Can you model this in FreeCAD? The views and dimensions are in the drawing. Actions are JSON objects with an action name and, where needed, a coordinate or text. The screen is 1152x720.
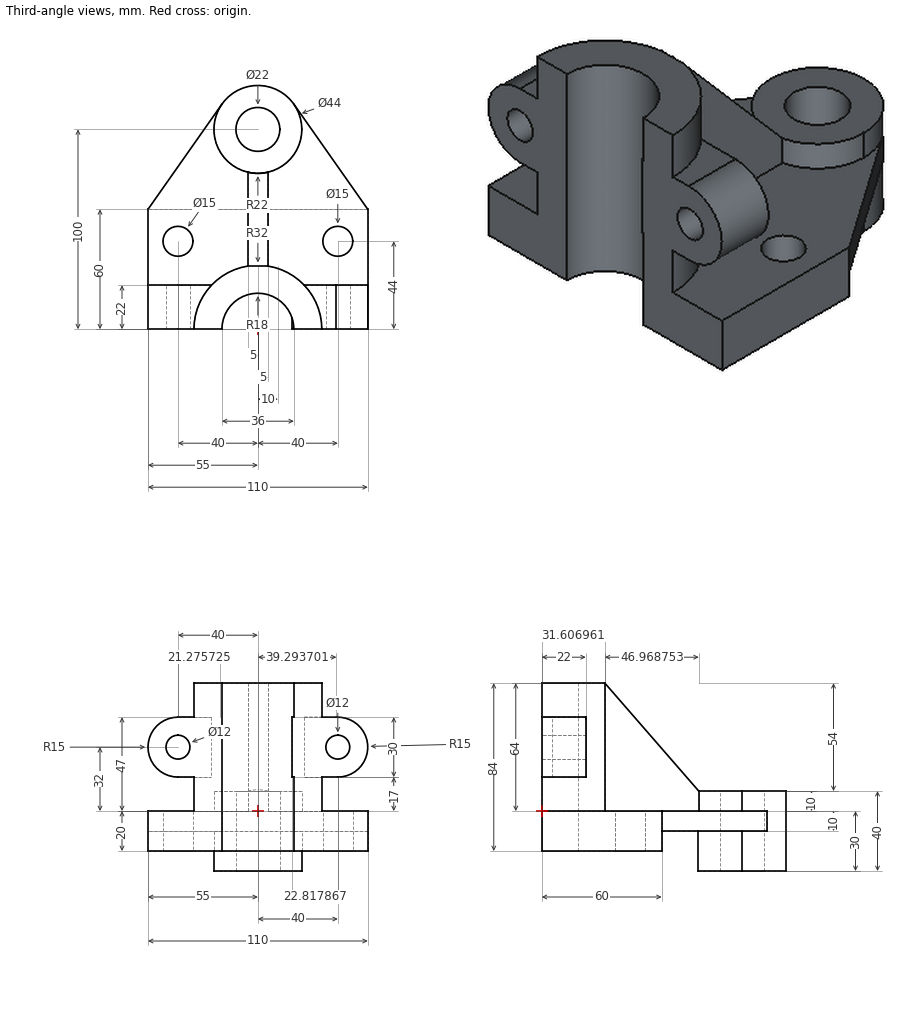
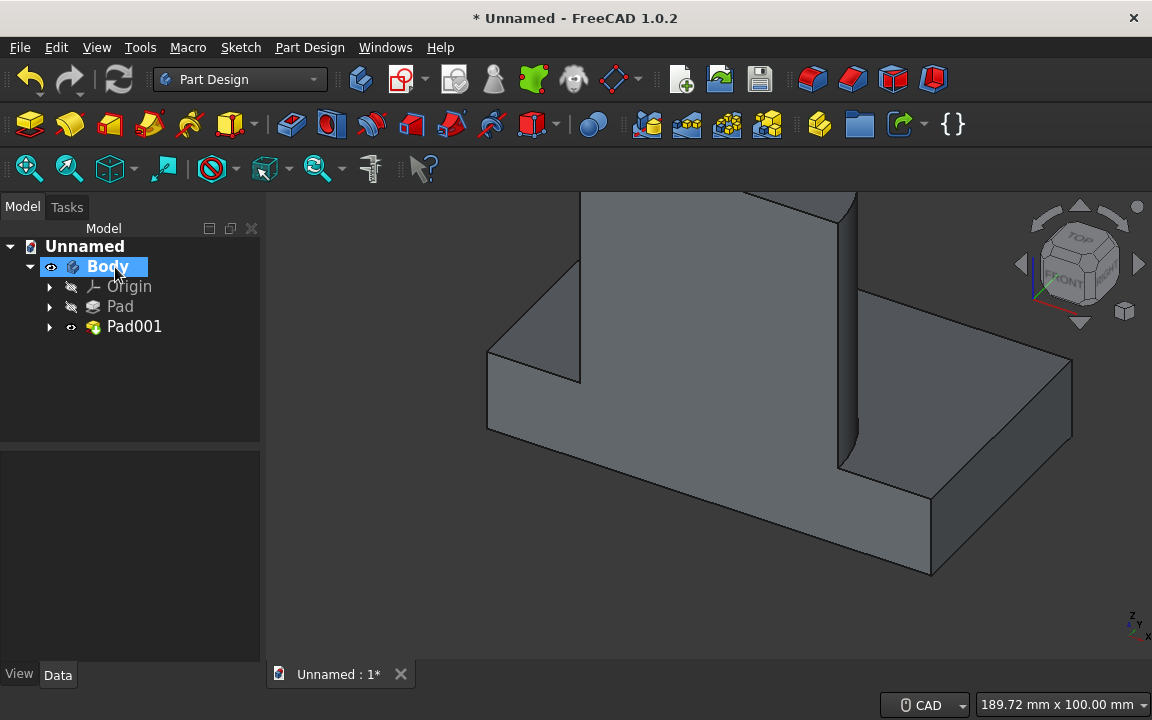
{"action": "left_click", "coordinate": [30, 170]}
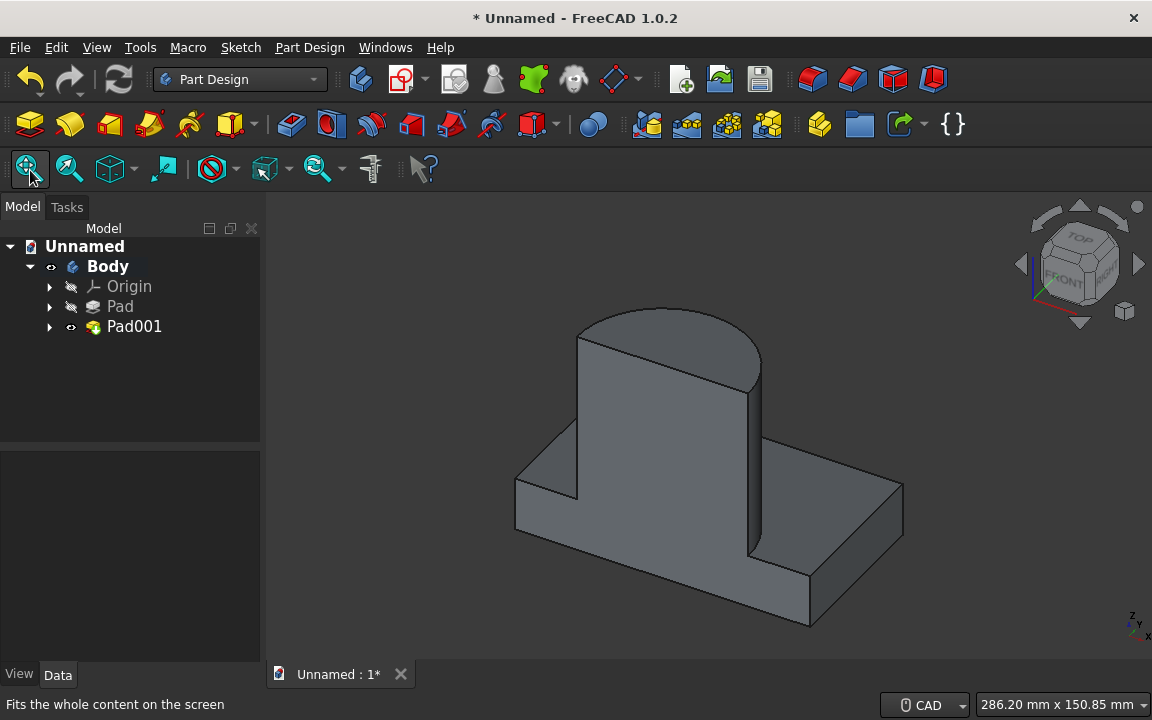
{"action": "left_click", "coordinate": [687, 340]}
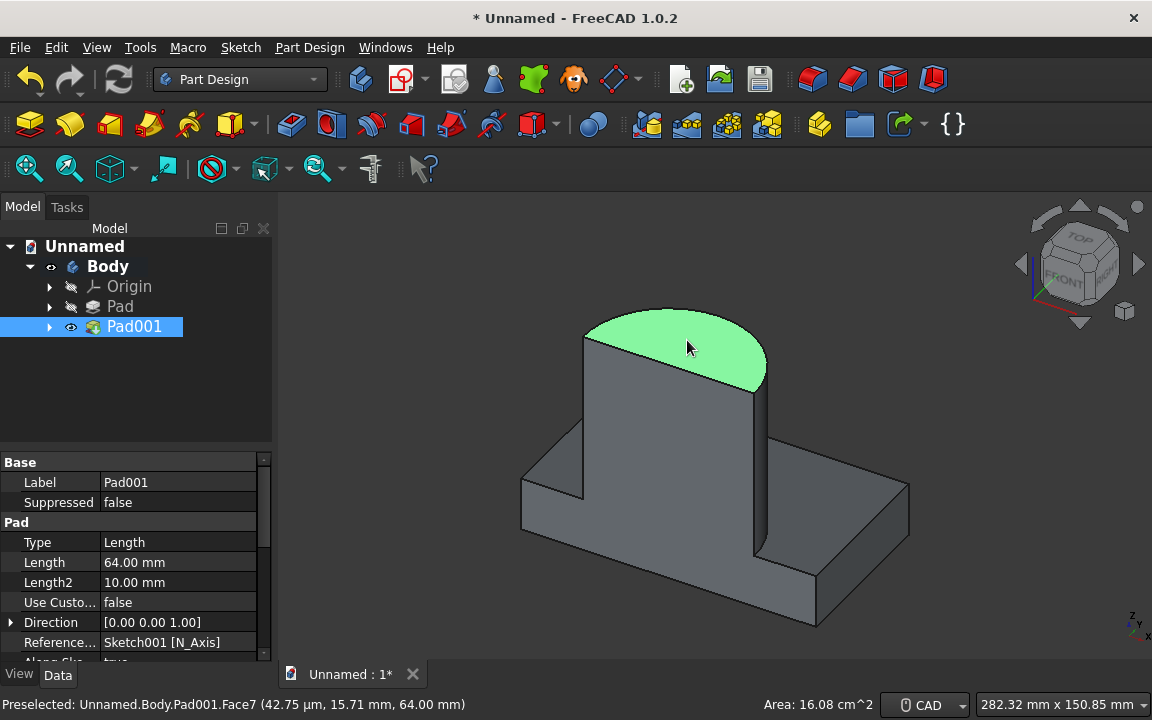
{"action": "left_click", "coordinate": [402, 80]}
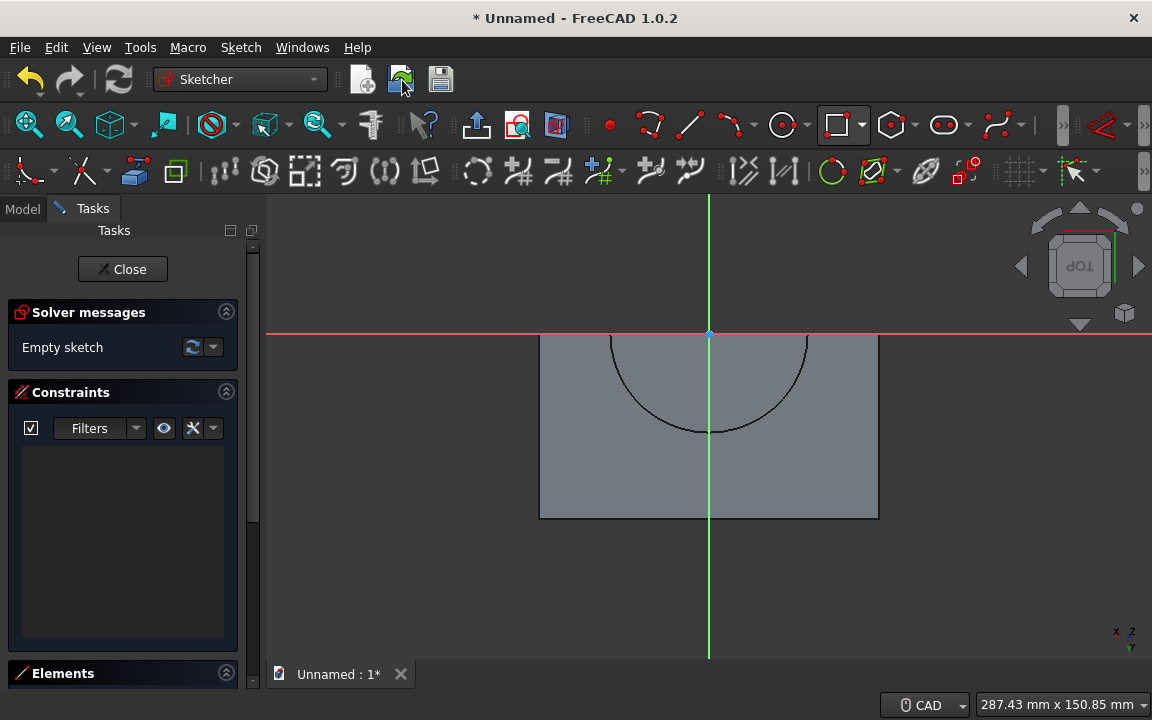
{"action": "scroll", "coordinate": [731, 341], "scroll_direction": "up", "scroll_amount": 7}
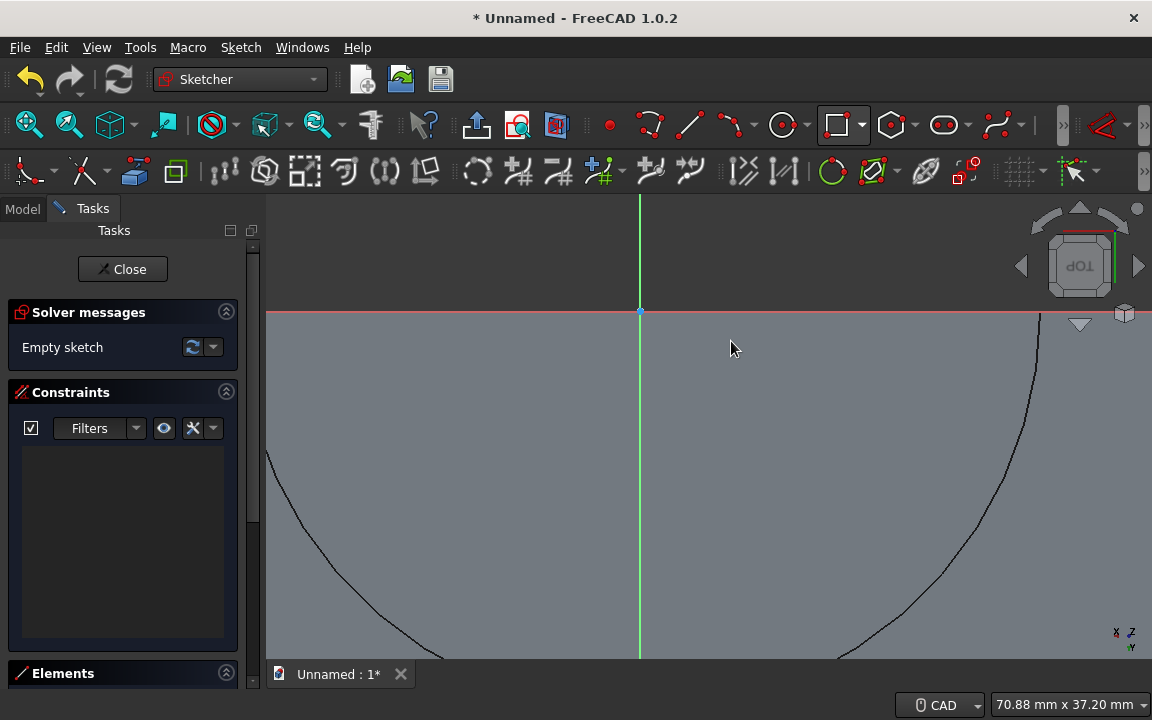
{"action": "left_click", "coordinate": [690, 126]}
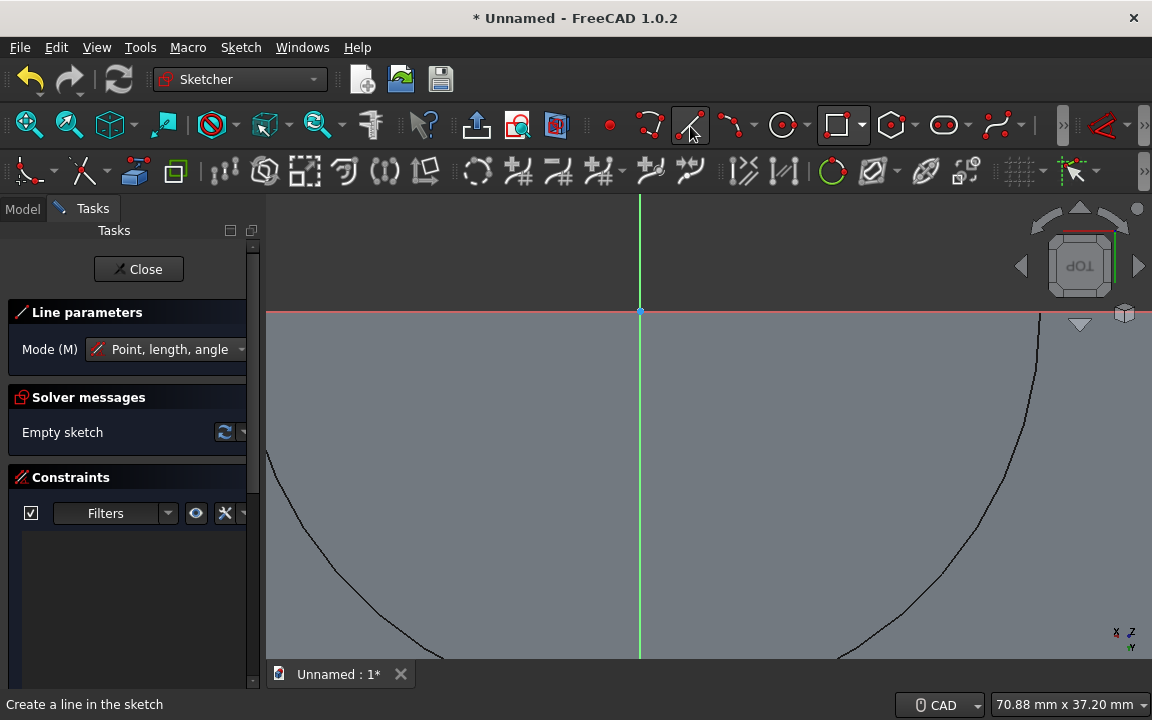
{"action": "left_click", "coordinate": [865, 312]}
{"action": "left_click", "coordinate": [415, 321]}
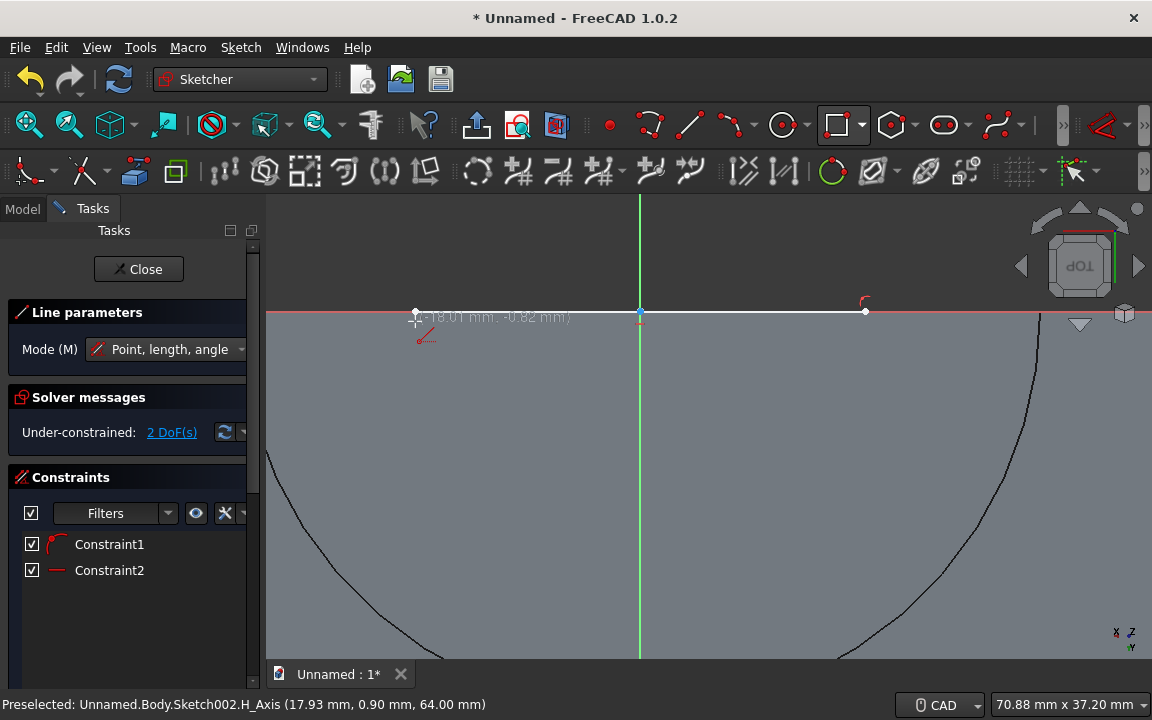
{"action": "left_click", "coordinate": [730, 126]}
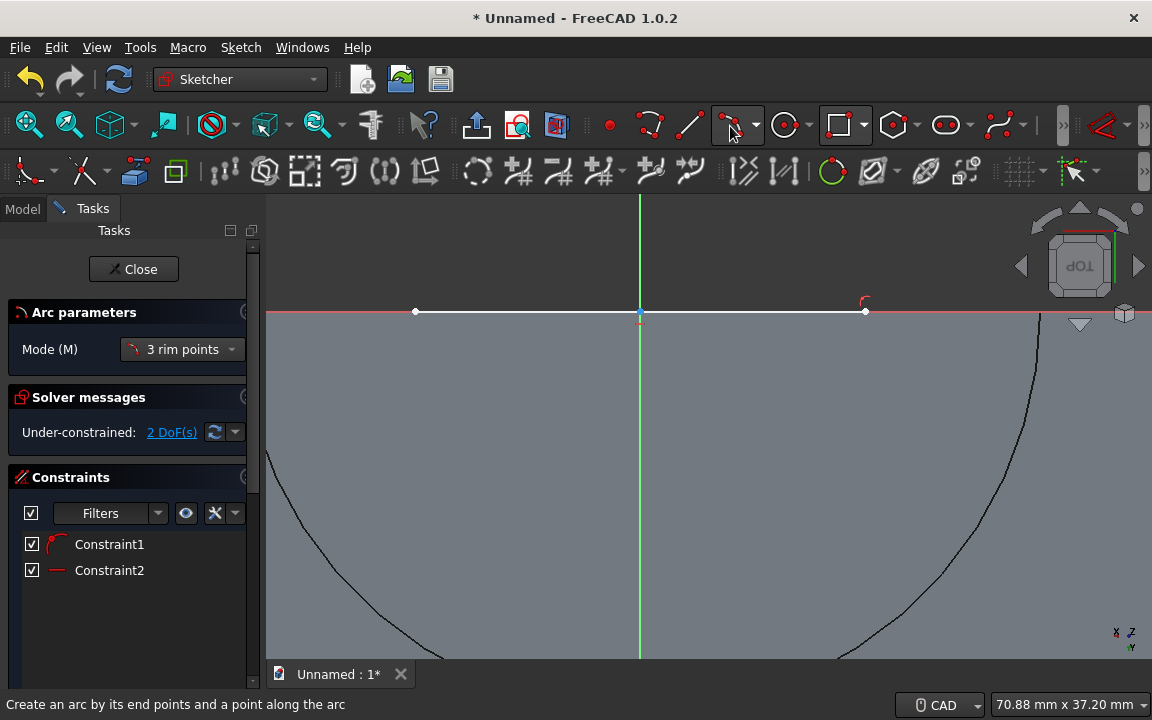
{"action": "left_click", "coordinate": [415, 321]}
{"action": "left_click", "coordinate": [865, 312]}
{"action": "left_click", "coordinate": [571, 526]}
{"action": "key", "text": "Escape"}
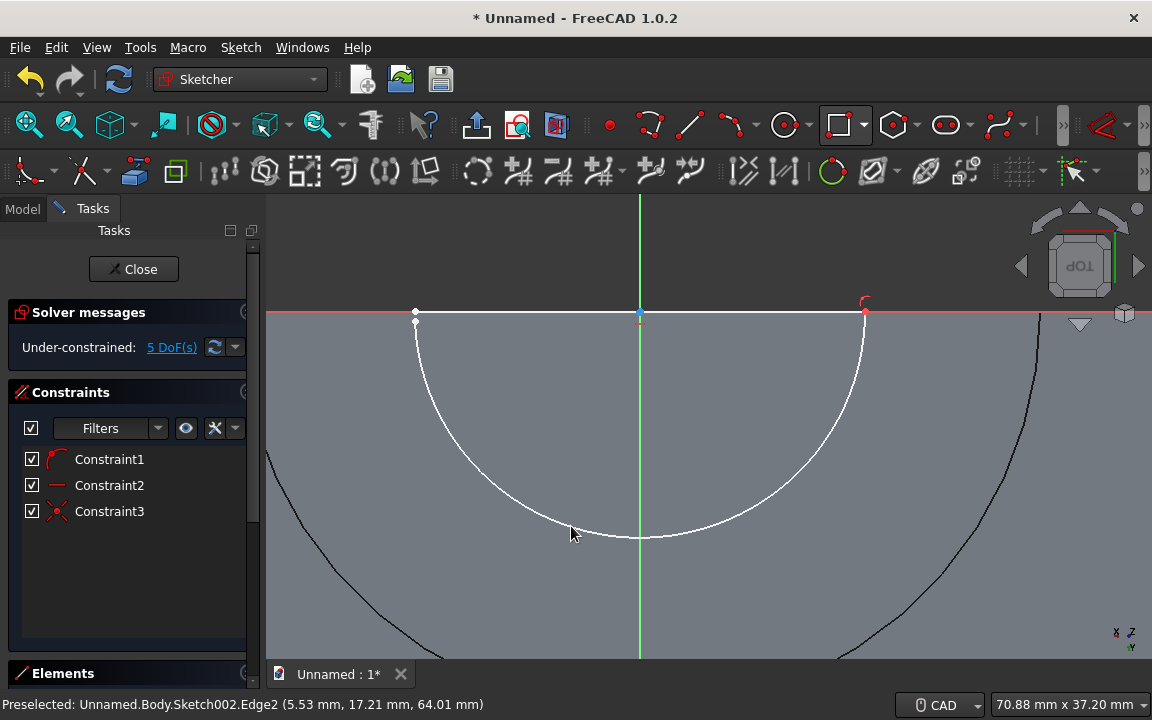
{"action": "left_click_drag", "start_coordinate": [630, 302], "coordinate": [650, 323]}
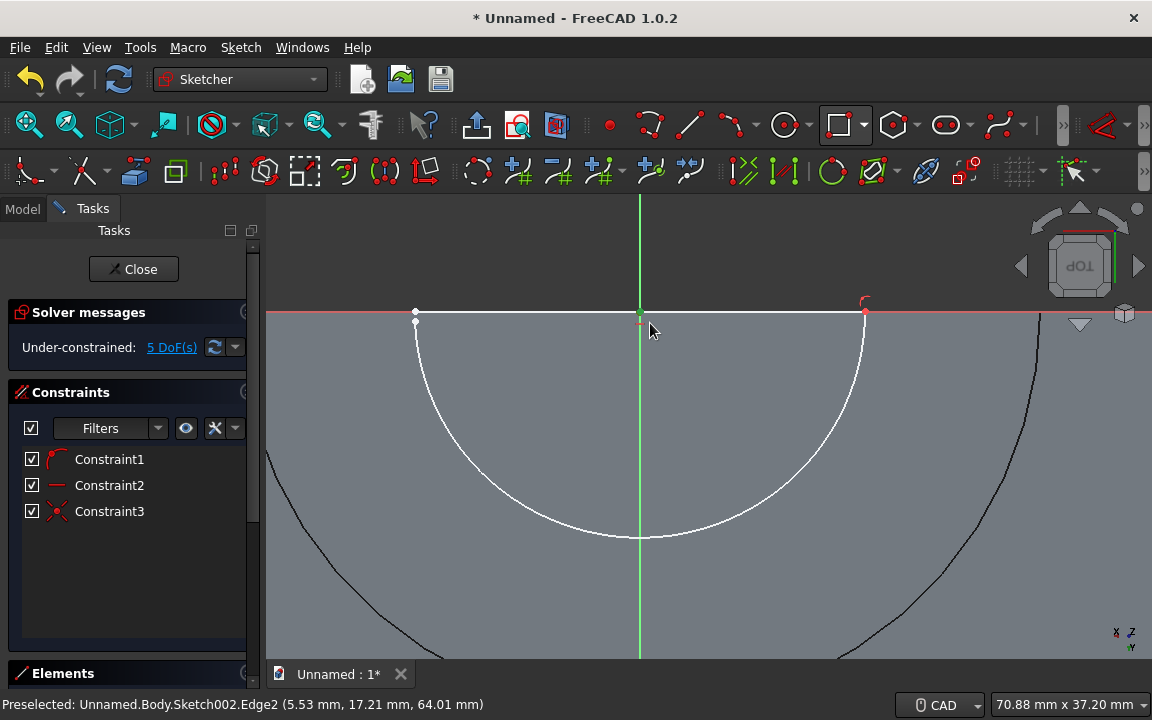
{"action": "key", "text": "c"}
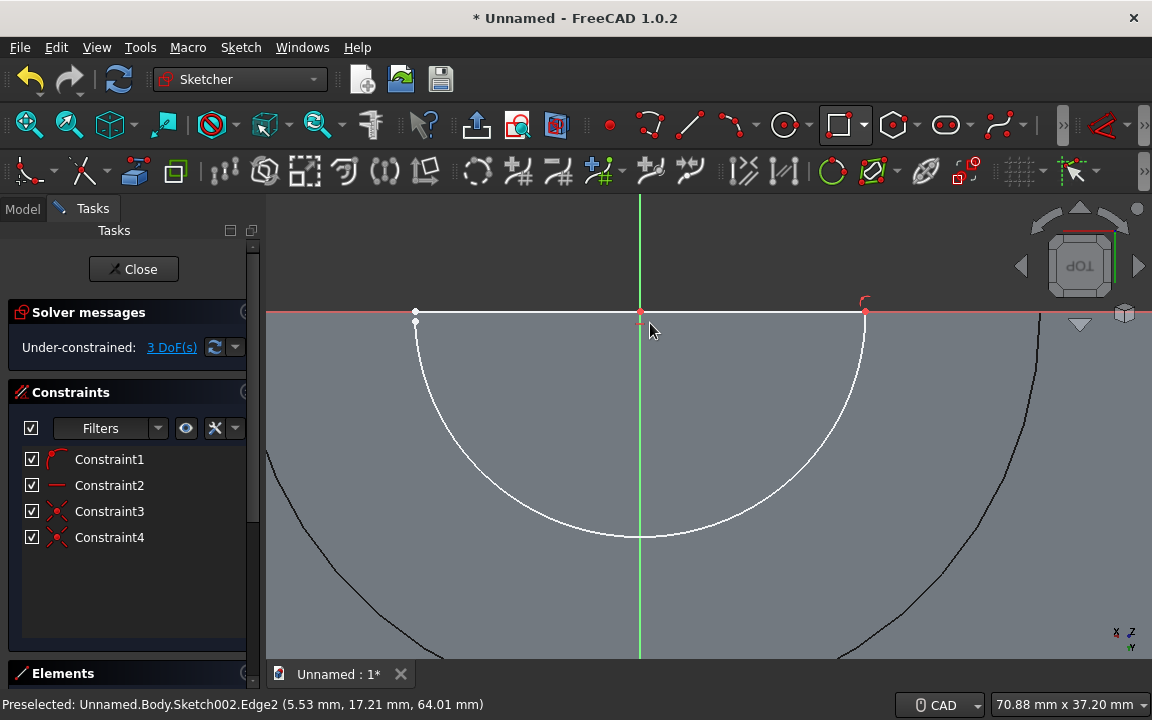
{"action": "left_click", "coordinate": [1102, 126]}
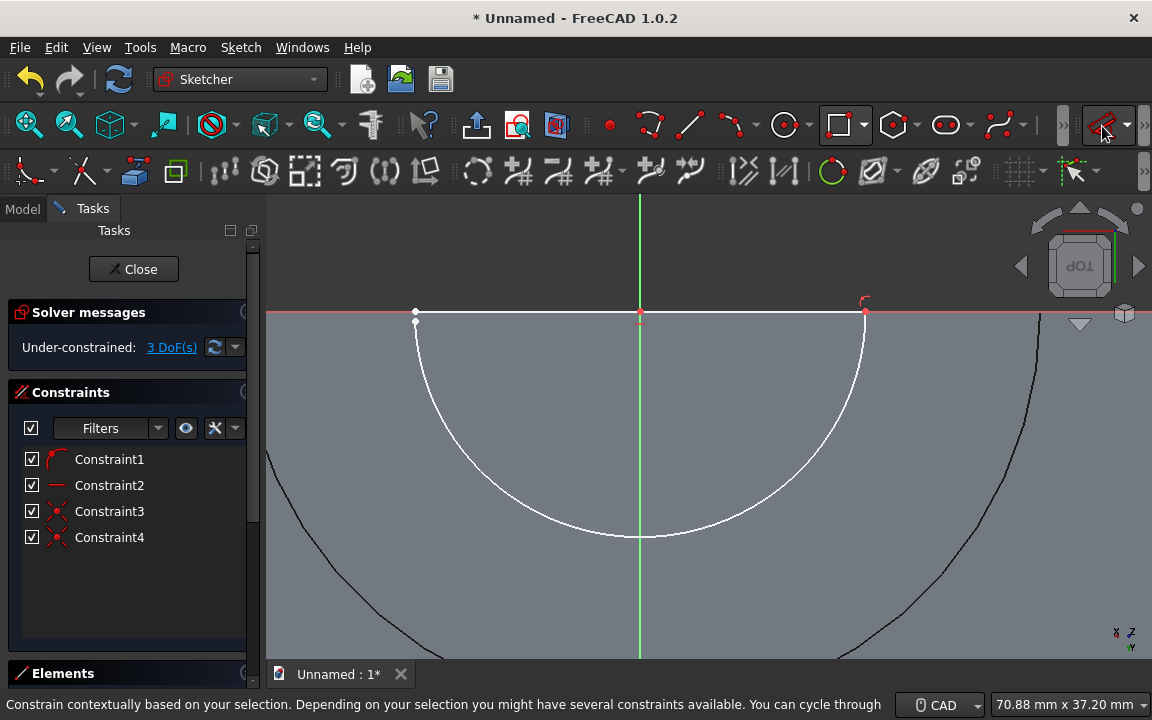
{"action": "left_click", "coordinate": [514, 498]}
{"action": "left_click", "coordinate": [496, 524]}